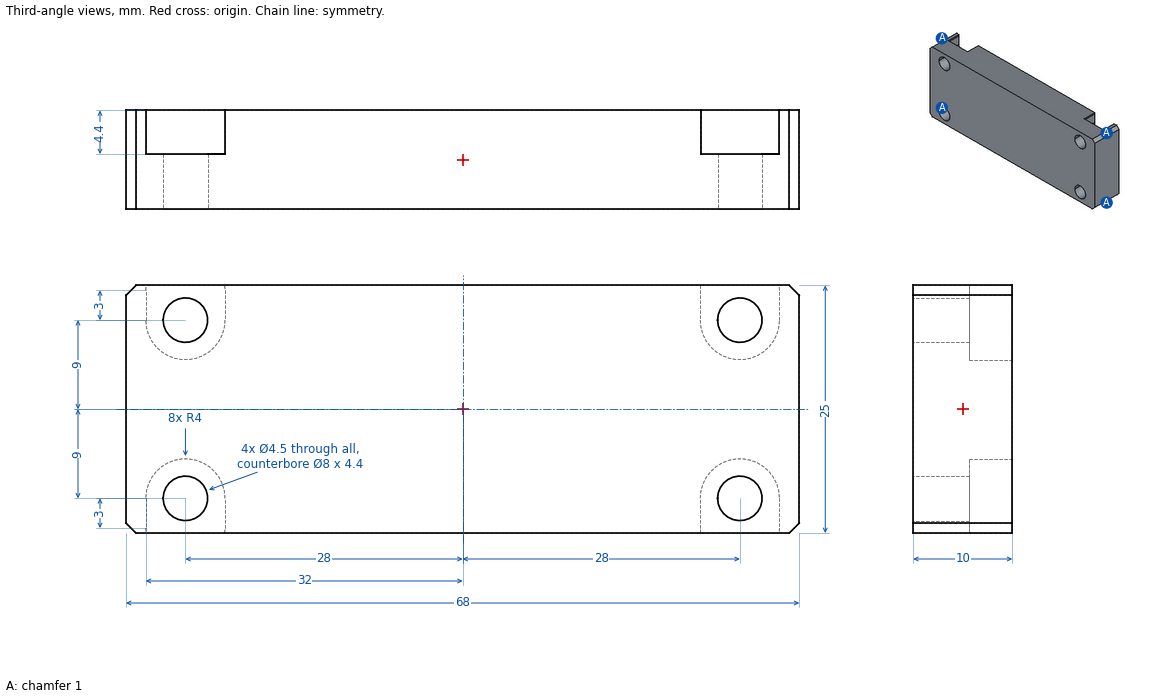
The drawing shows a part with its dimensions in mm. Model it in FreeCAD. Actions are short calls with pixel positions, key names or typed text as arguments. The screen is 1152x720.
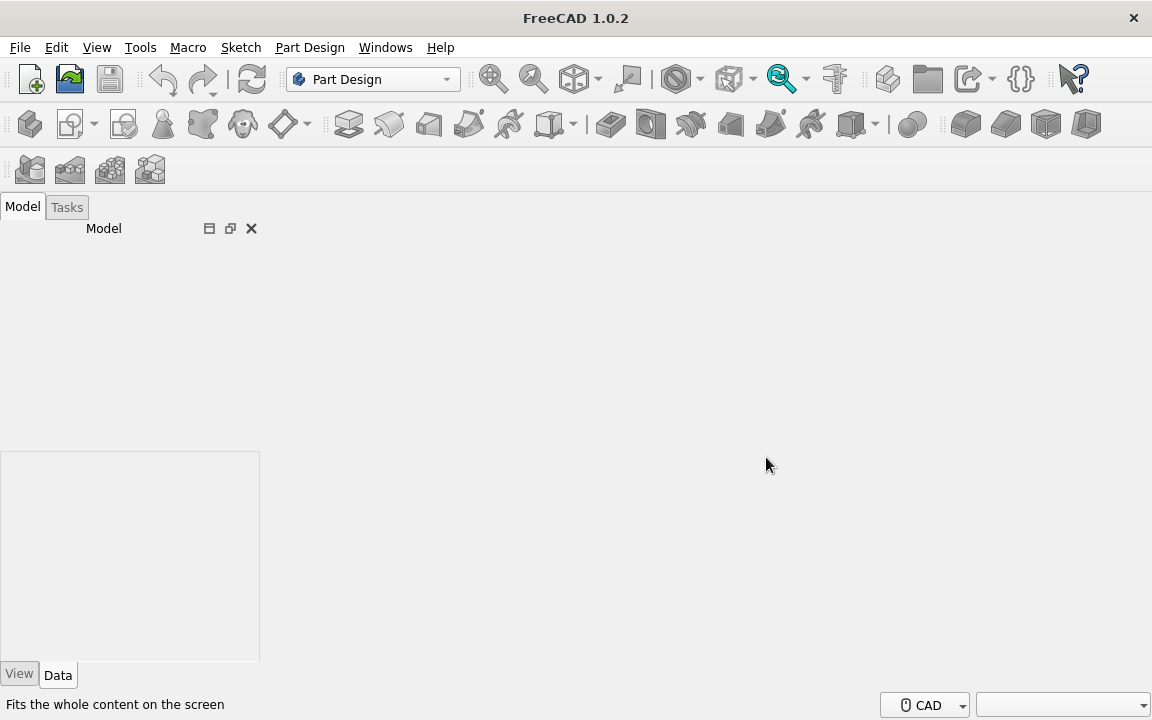
click(30, 80)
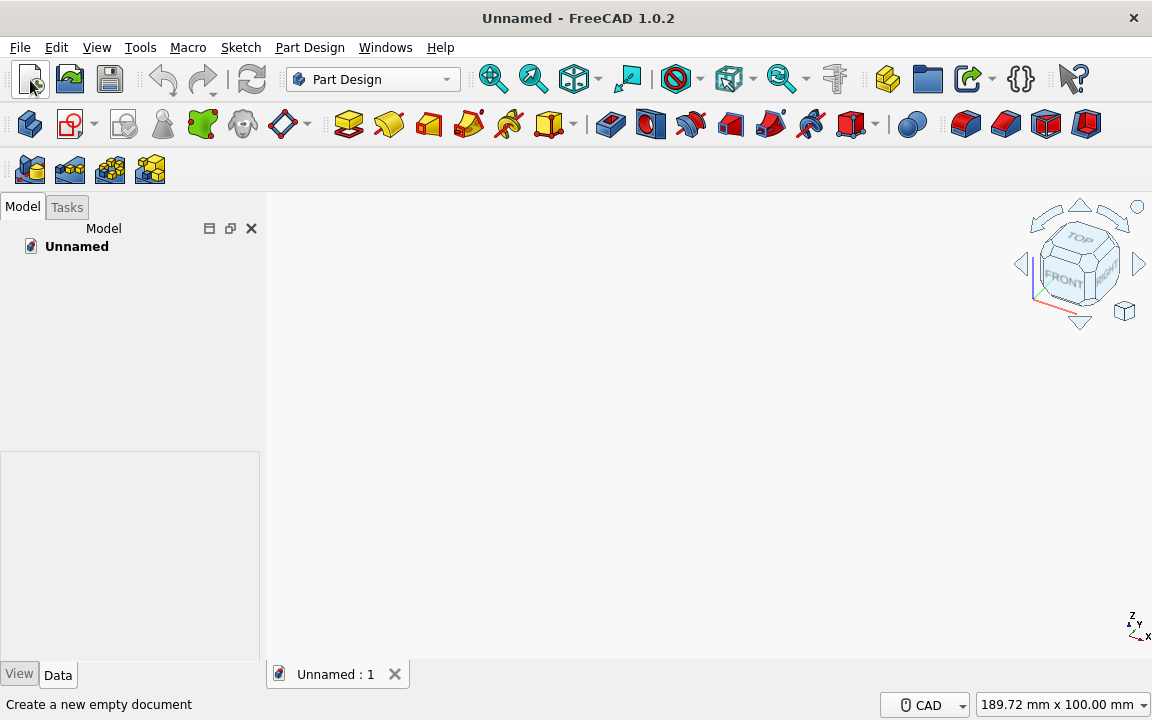
click(70, 124)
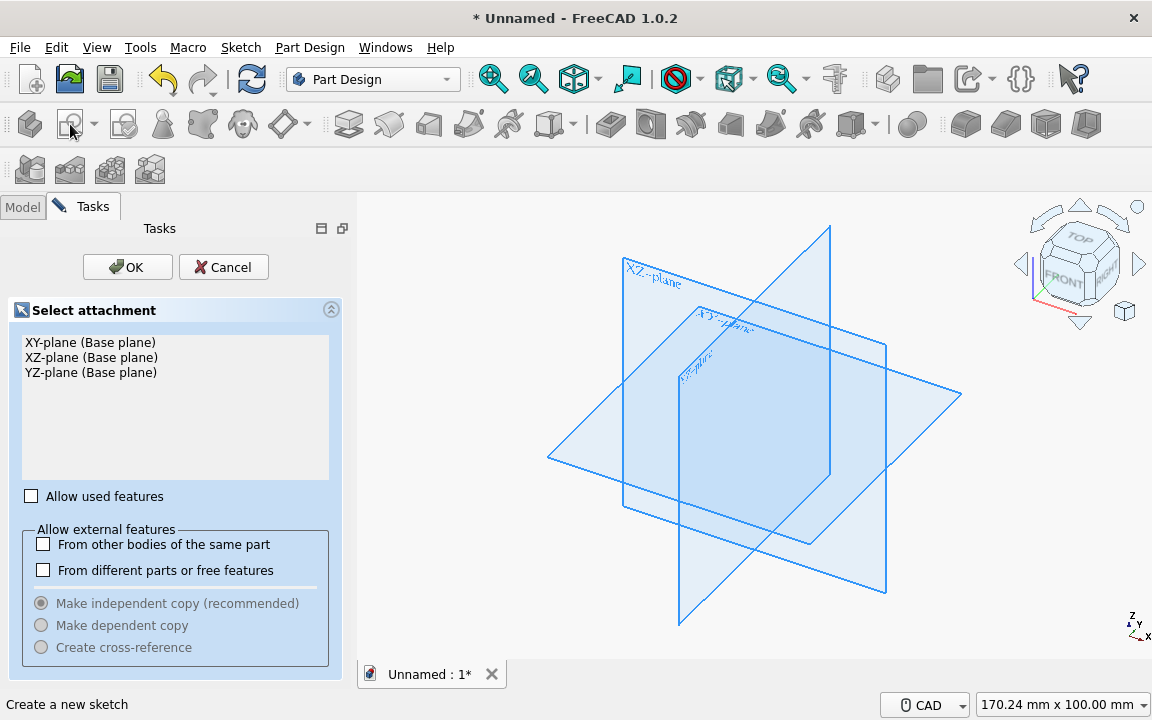
click(82, 358)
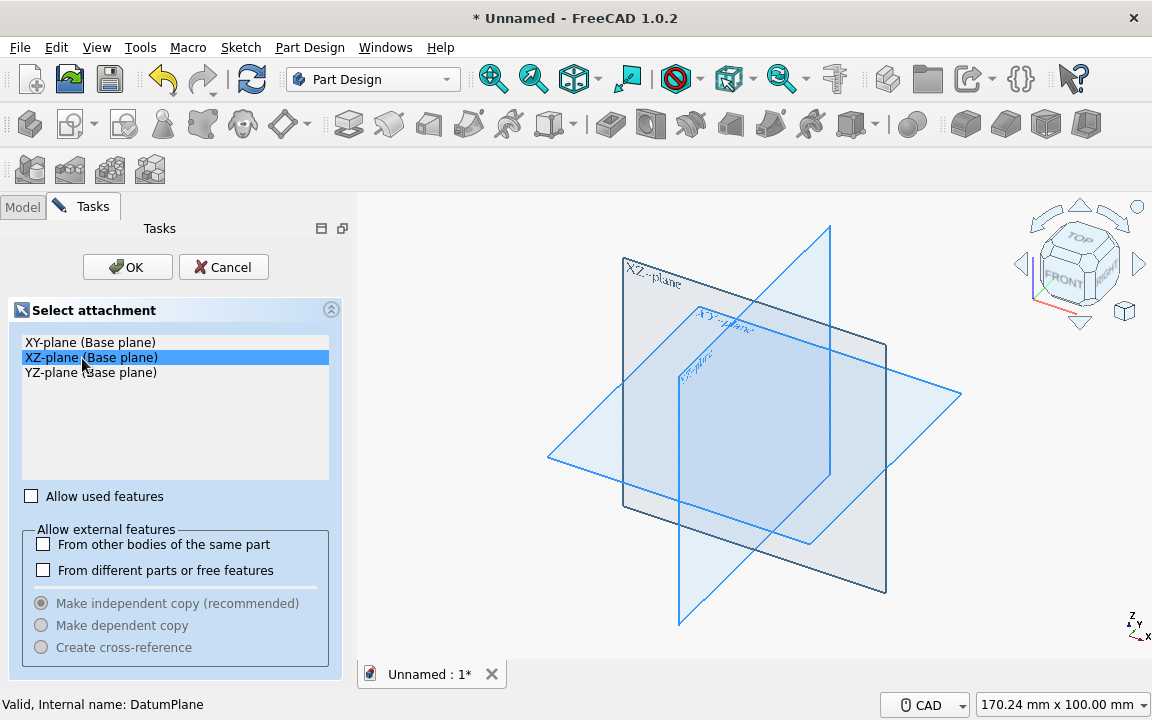
click(128, 267)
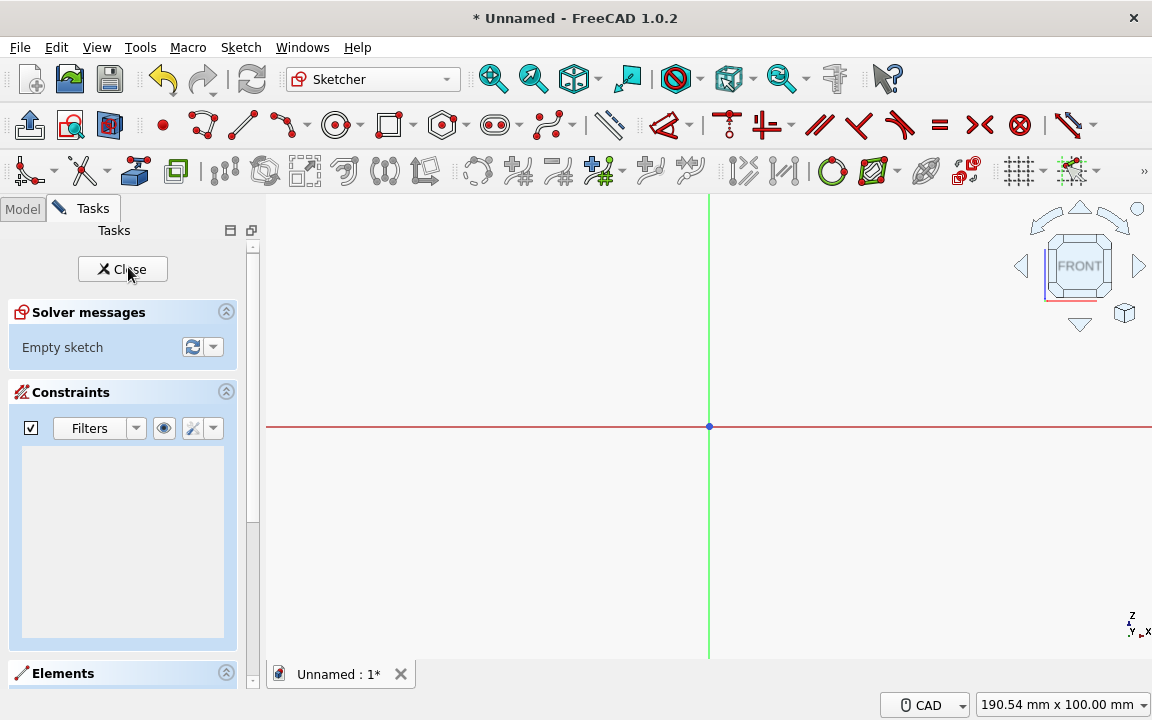
scroll(848, 426, up, 2)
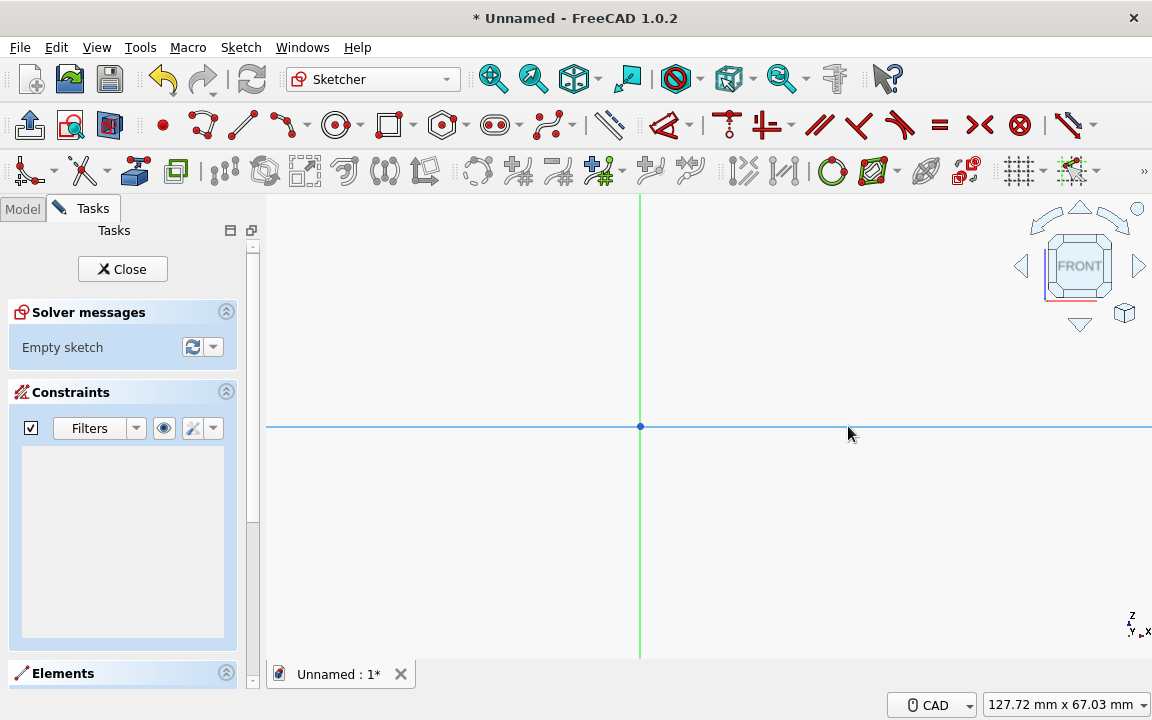
key(g)
key(v)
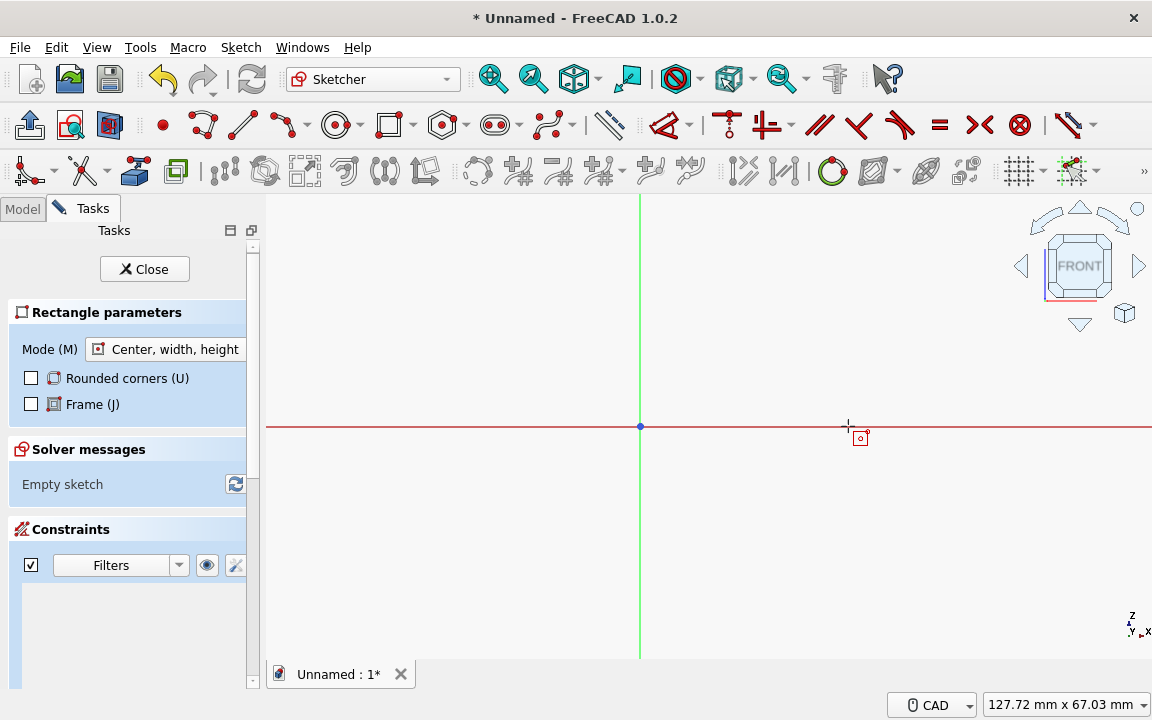
click(640, 426)
click(876, 340)
key(Escape)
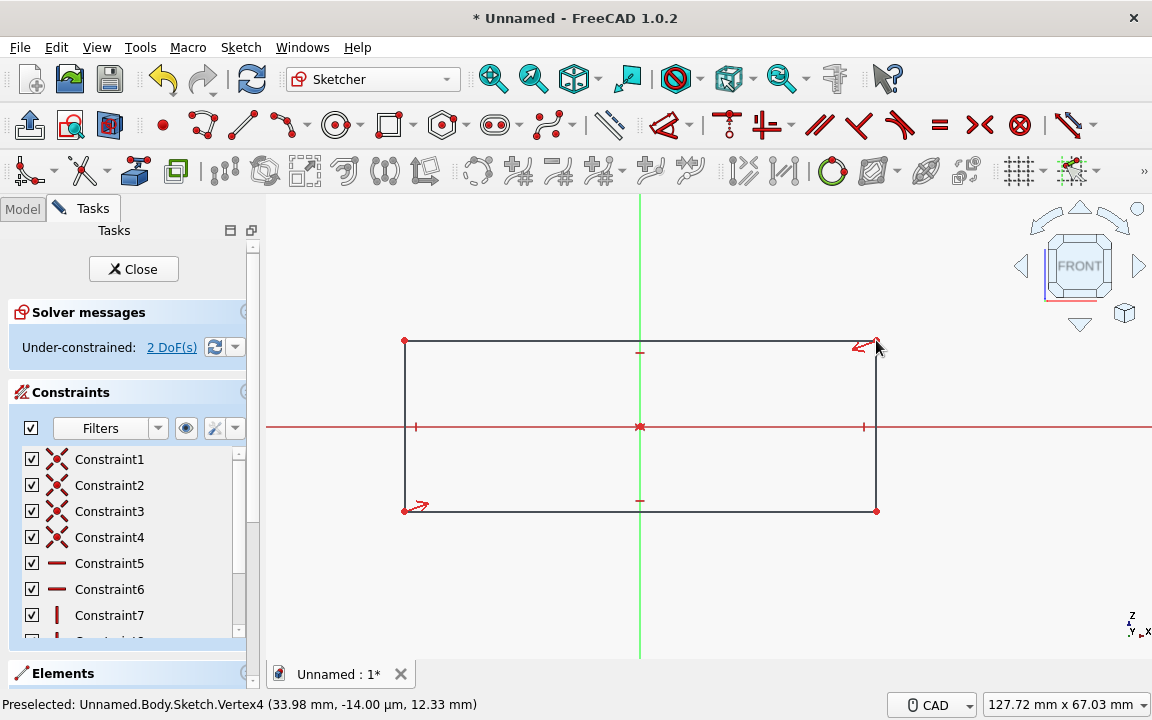
click(664, 126)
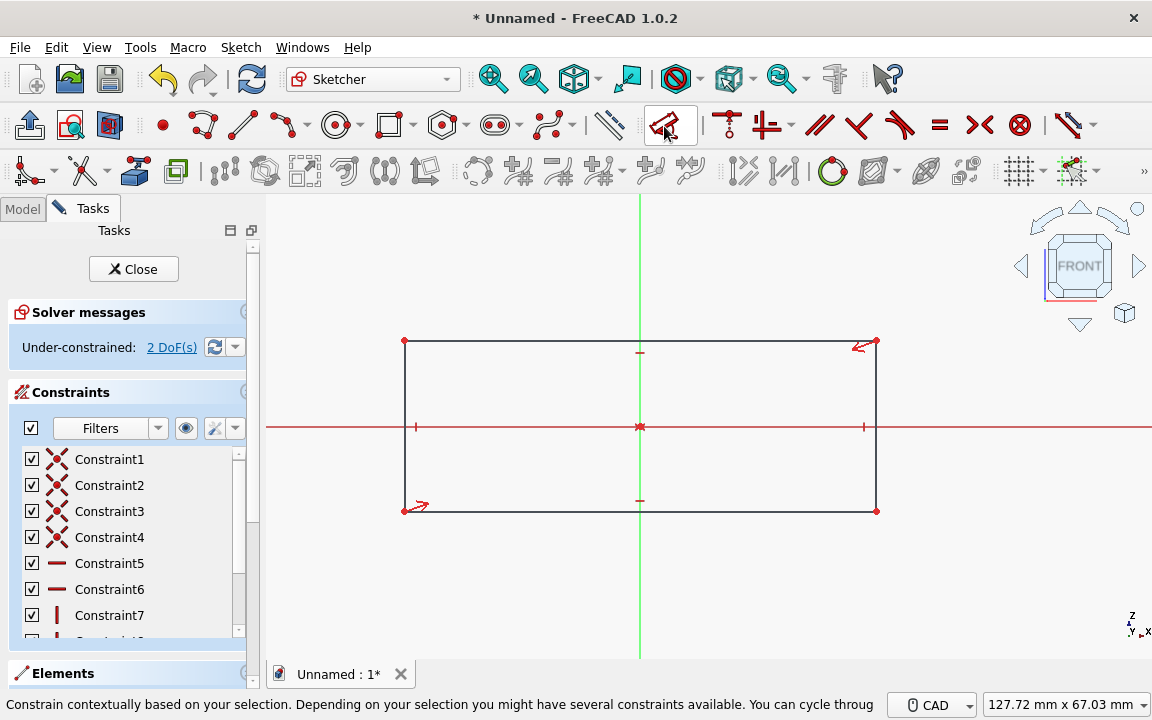
click(546, 512)
click(532, 546)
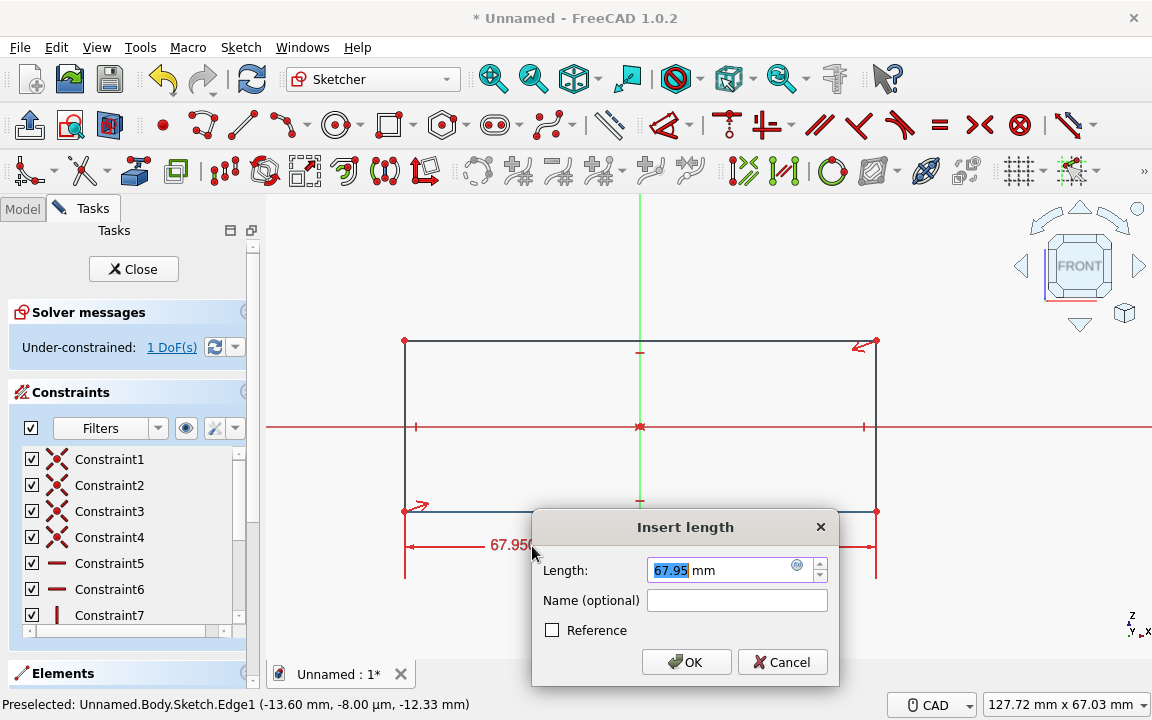
text(68)
key(Return)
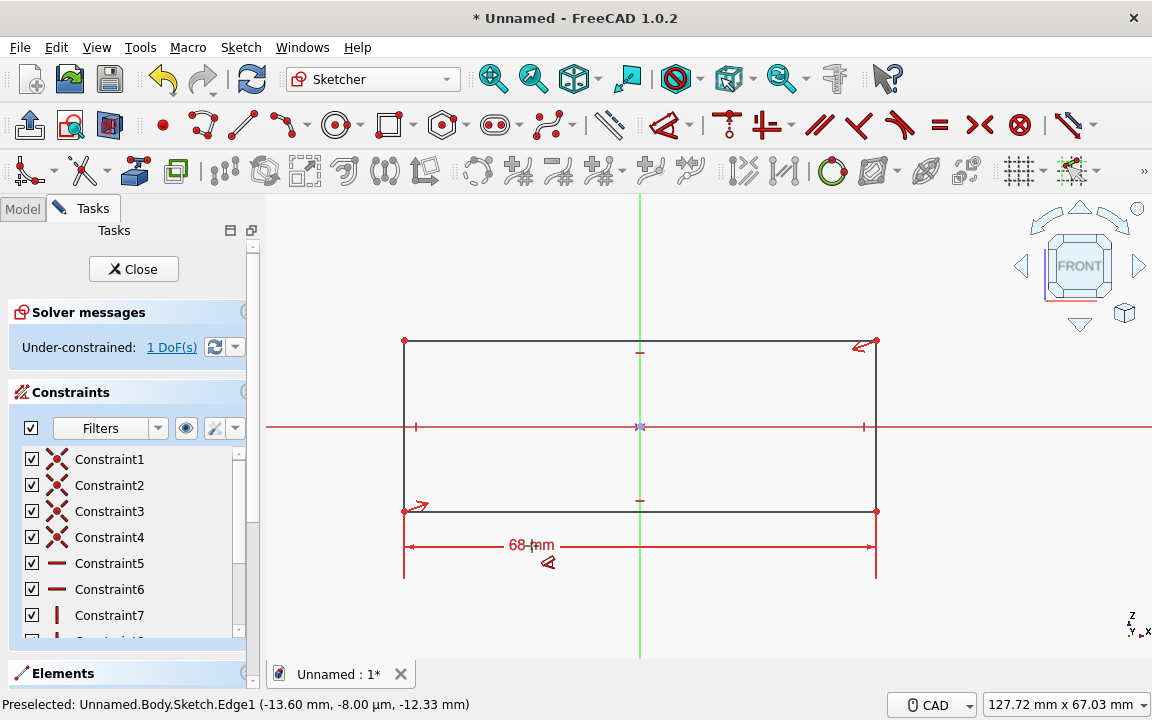
click(876, 461)
click(910, 387)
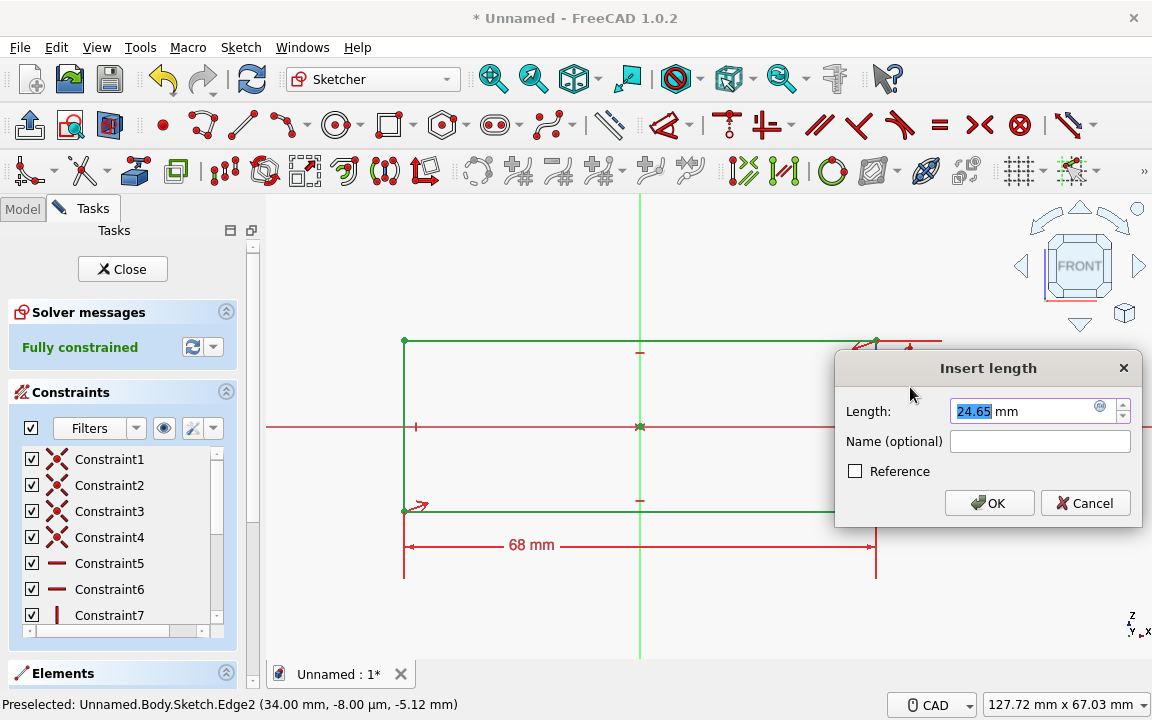
text(25)
key(Return)
key(Escape)